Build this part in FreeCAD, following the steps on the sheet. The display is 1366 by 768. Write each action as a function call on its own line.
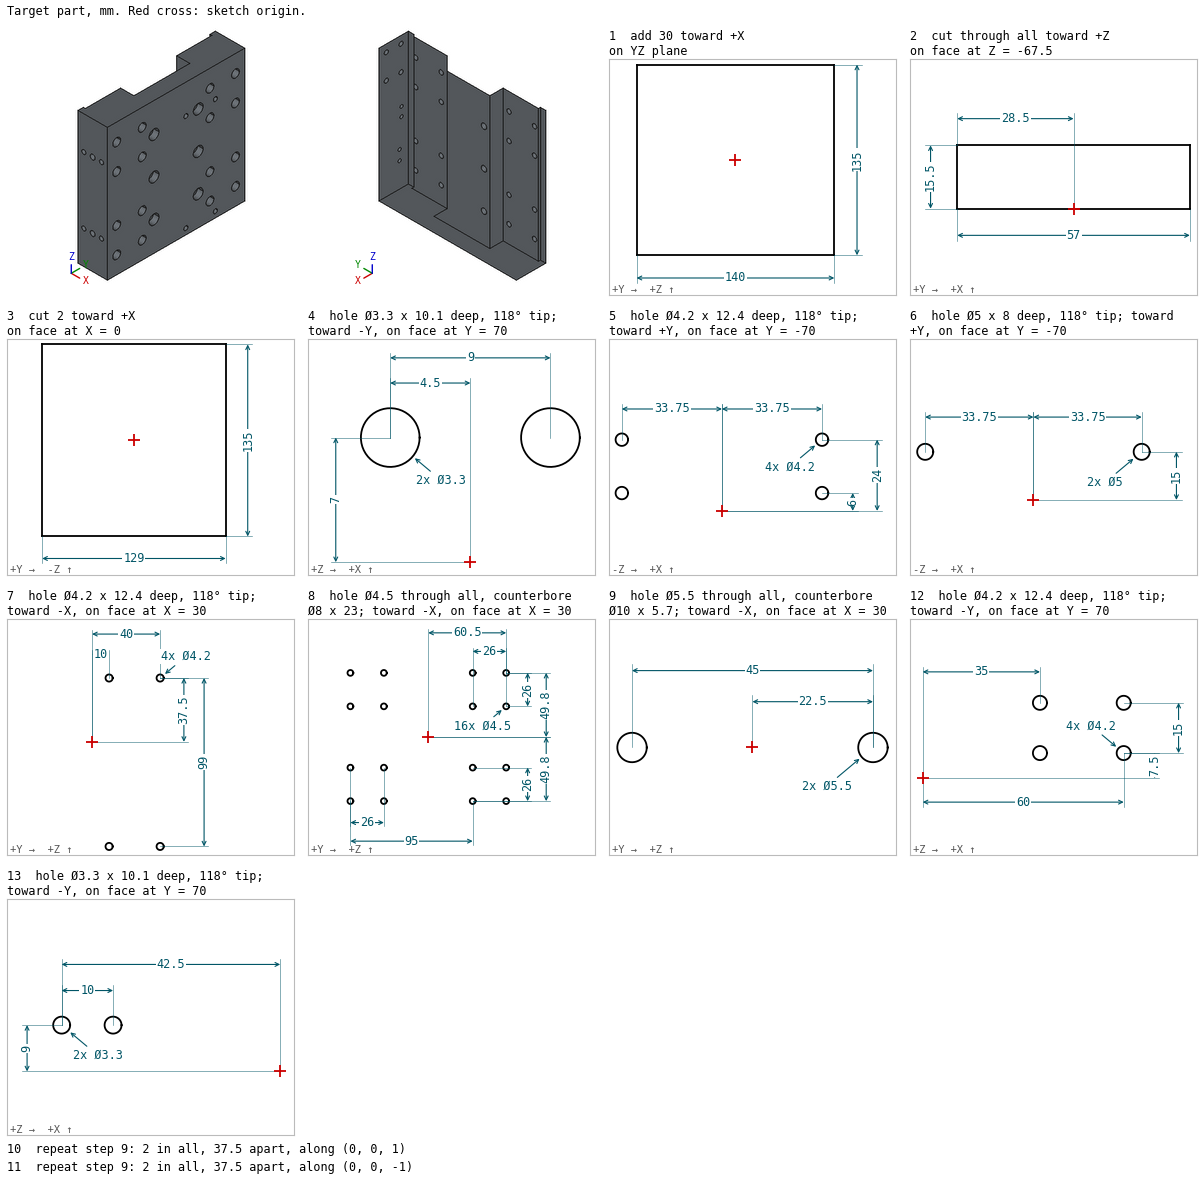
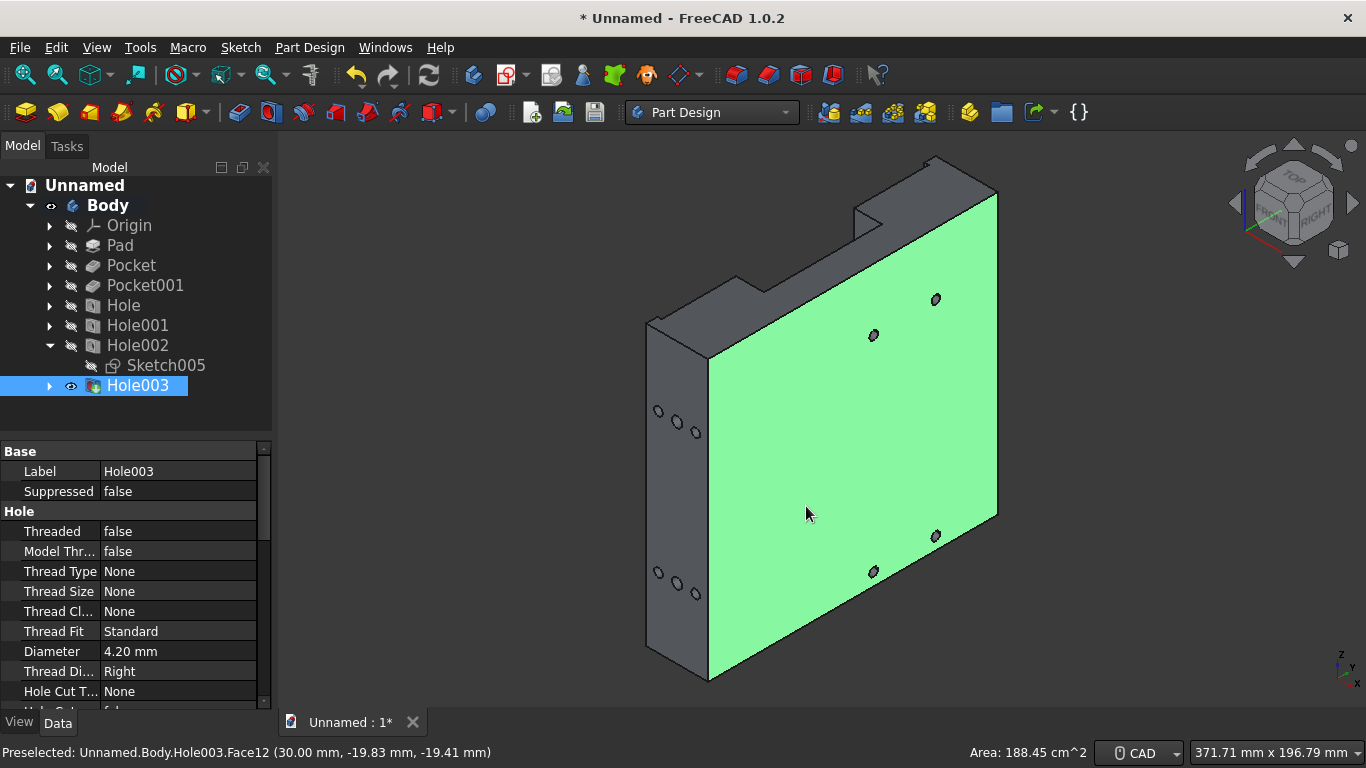
click(506, 76)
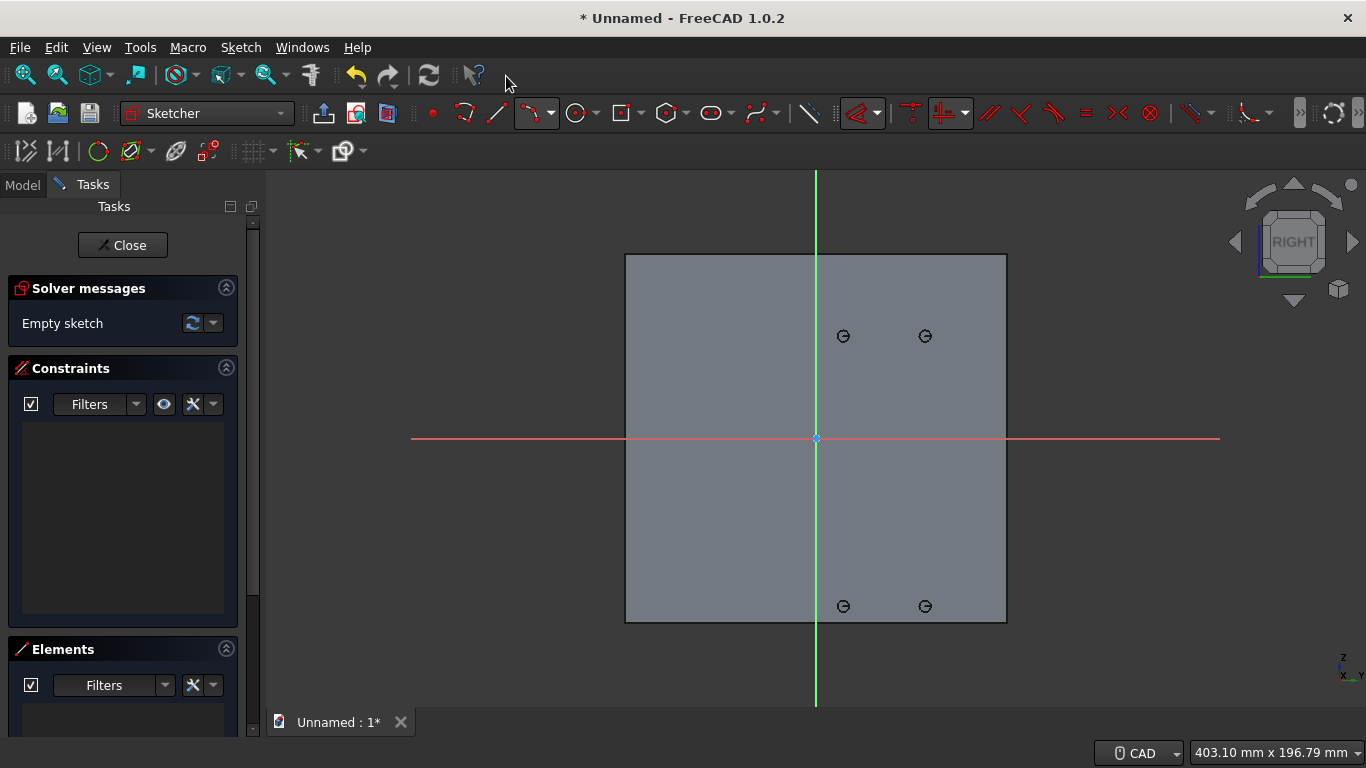
click(576, 114)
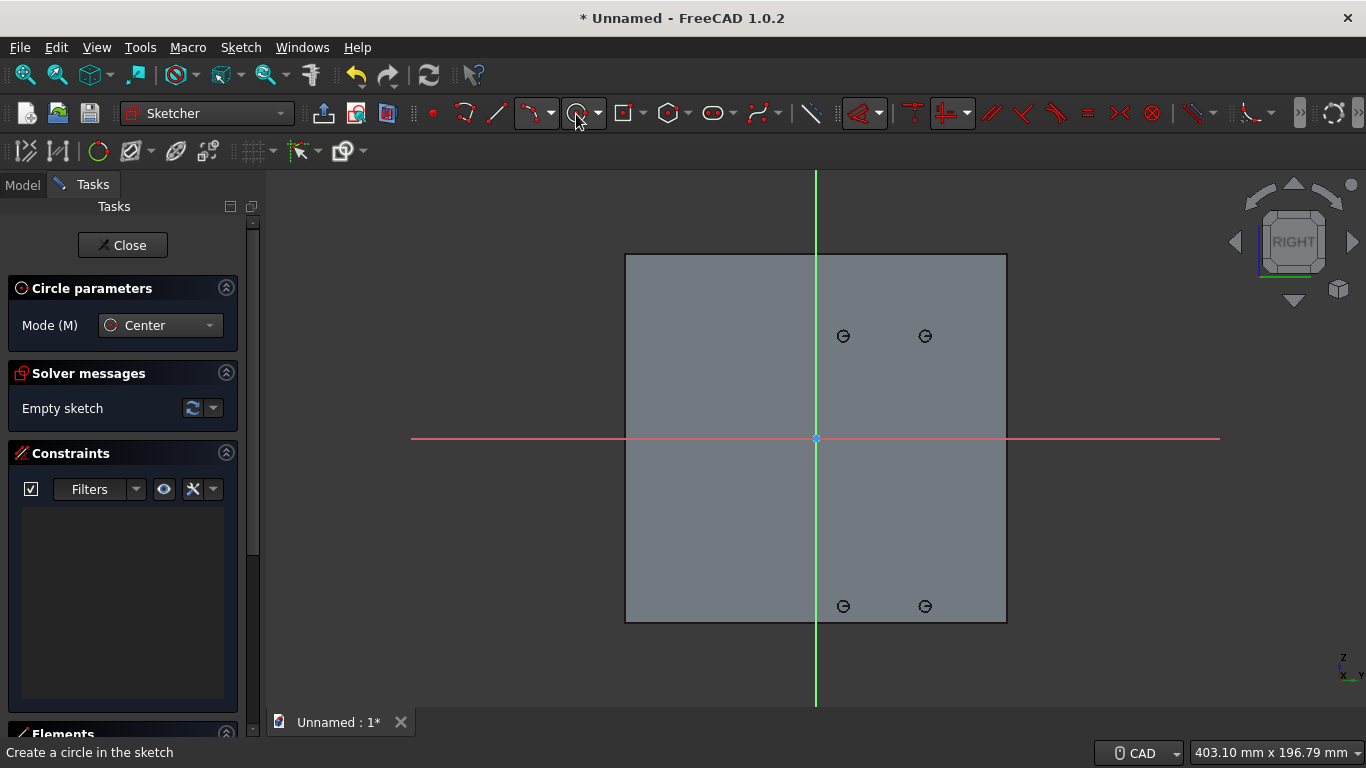
scroll(981, 303, up, 7)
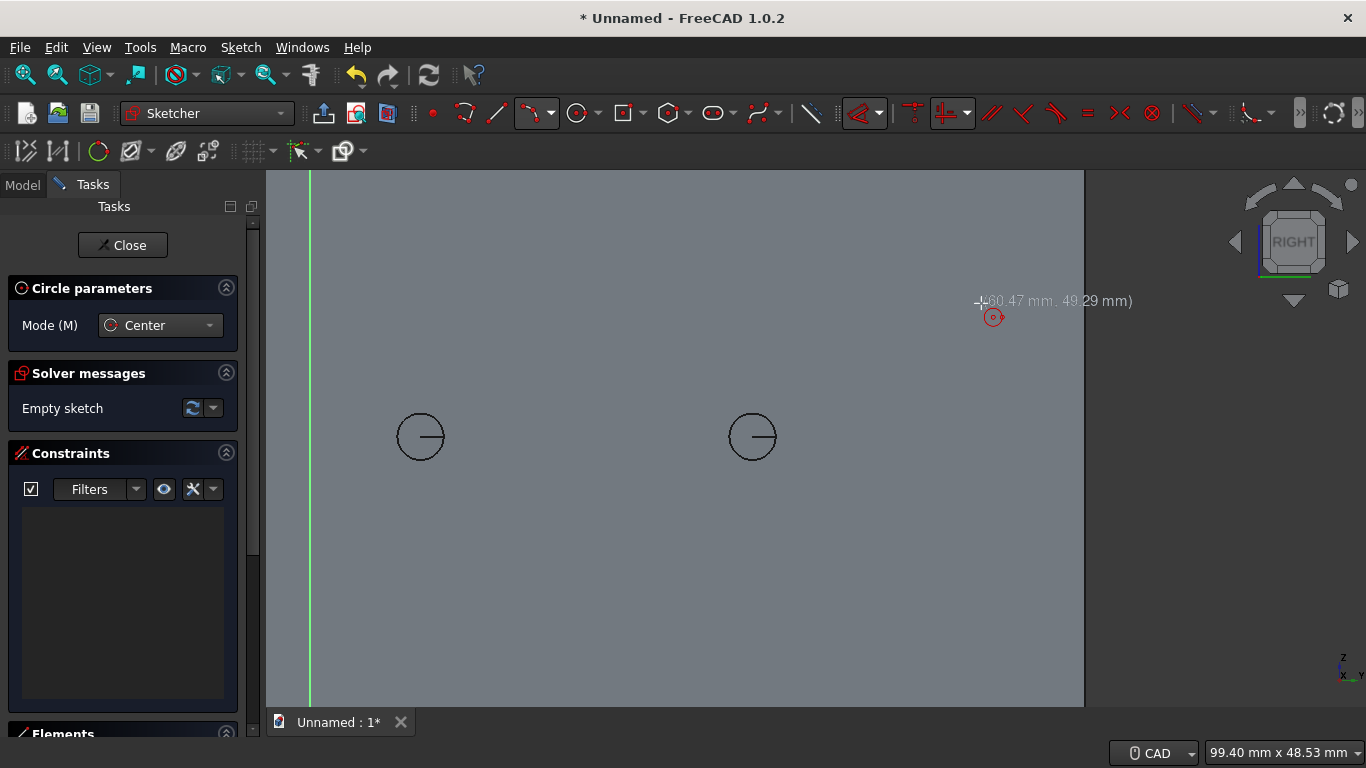
scroll(936, 260, down, 6)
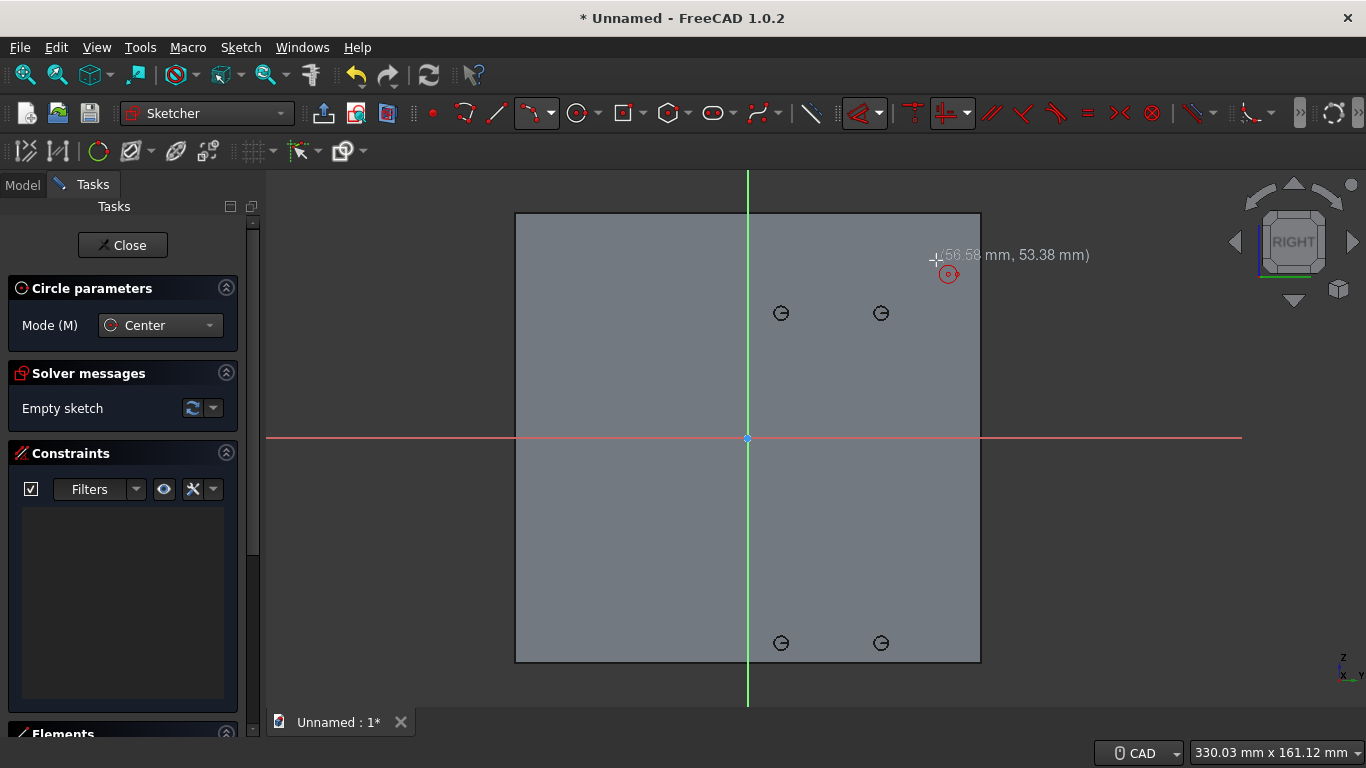
click(949, 272)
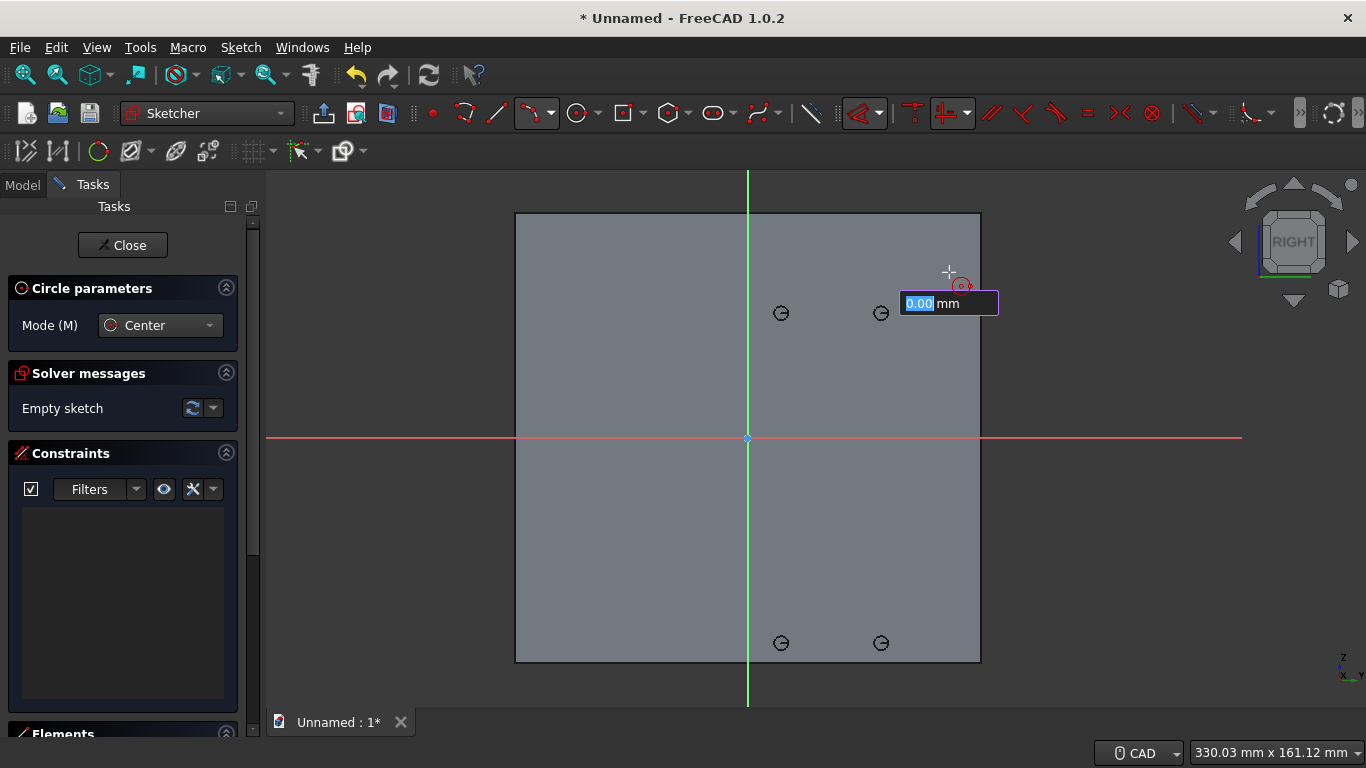
scroll(955, 267, up, 4)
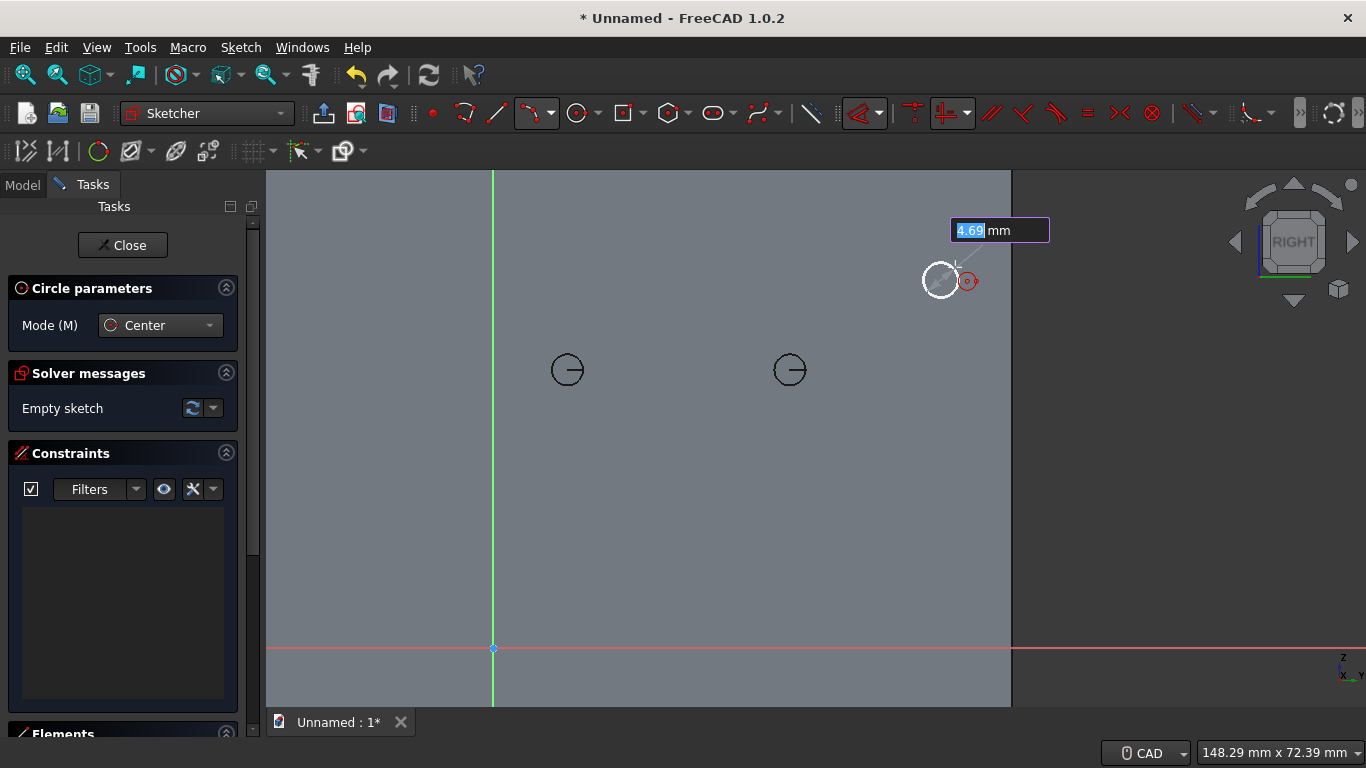
click(954, 267)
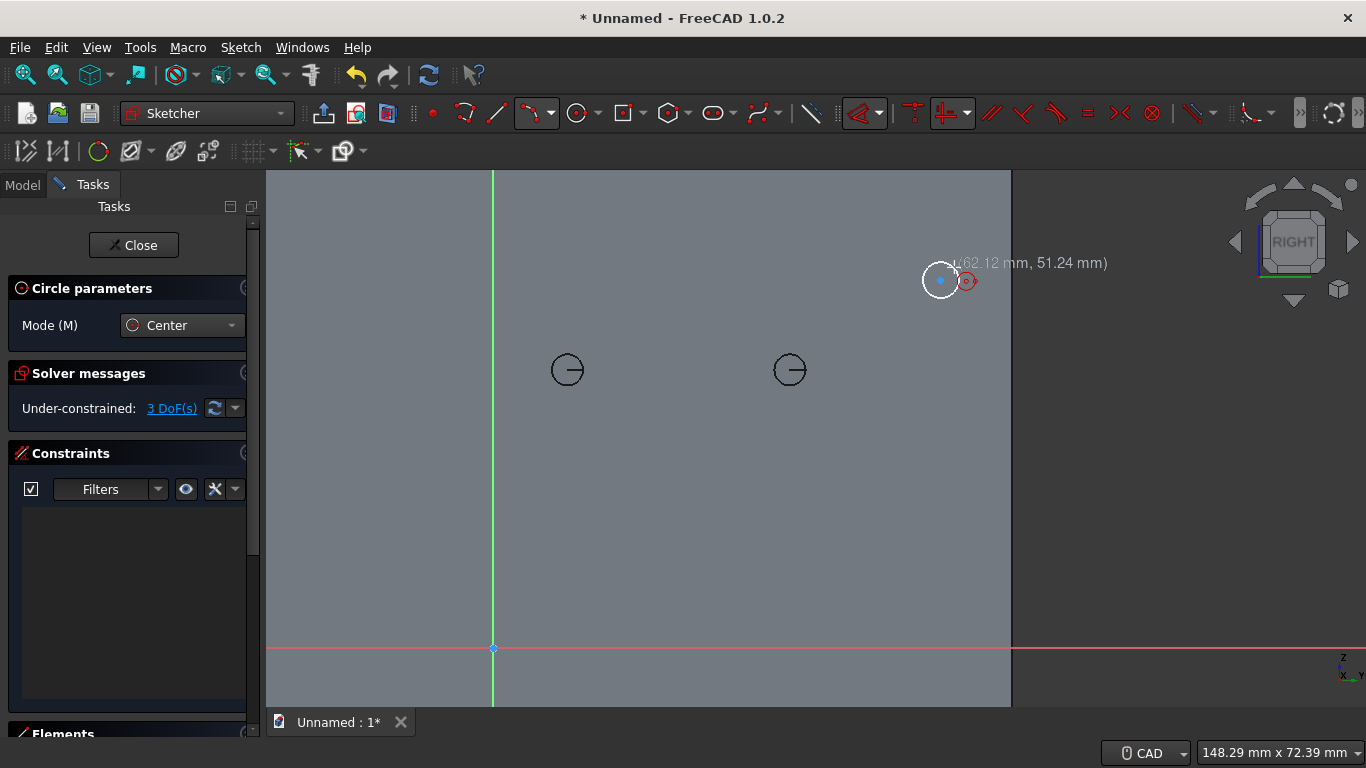
scroll(942, 472, up, 2)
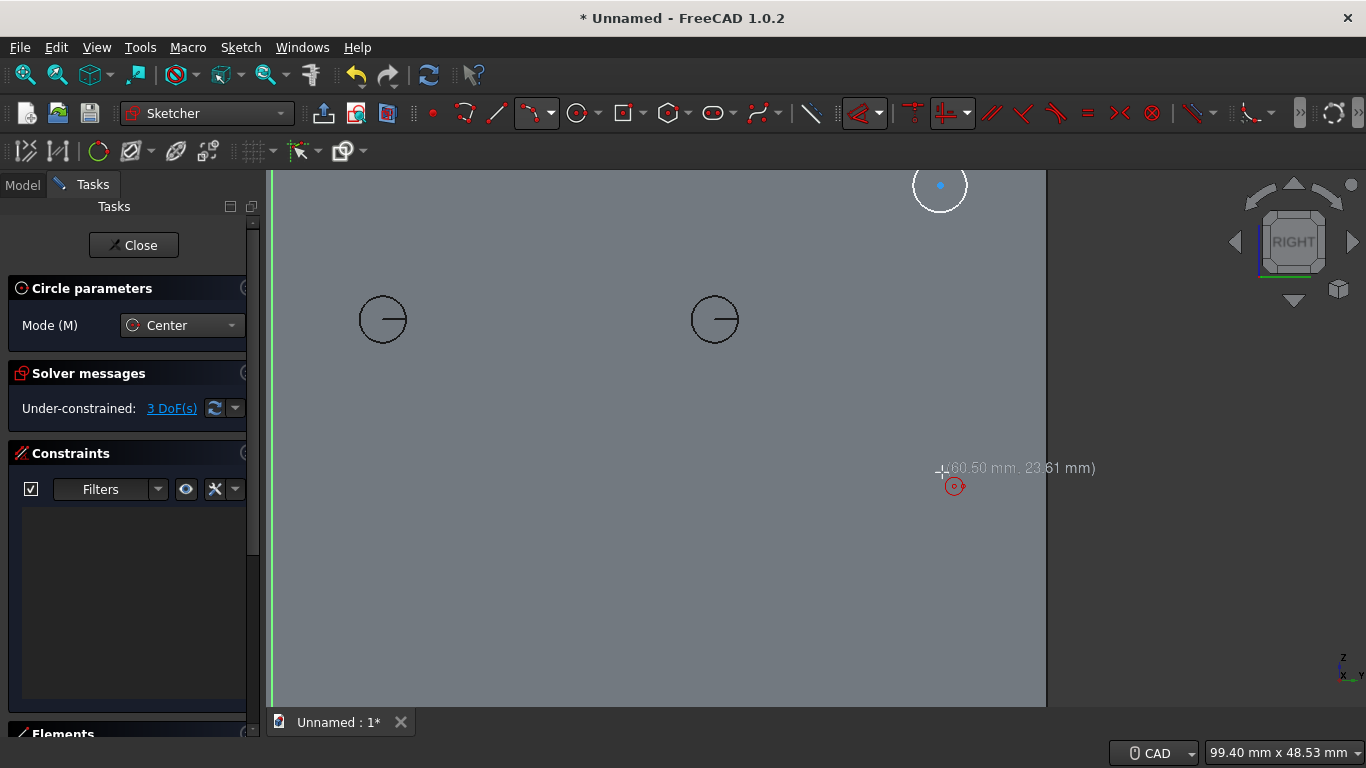
scroll(952, 311, down, 6)